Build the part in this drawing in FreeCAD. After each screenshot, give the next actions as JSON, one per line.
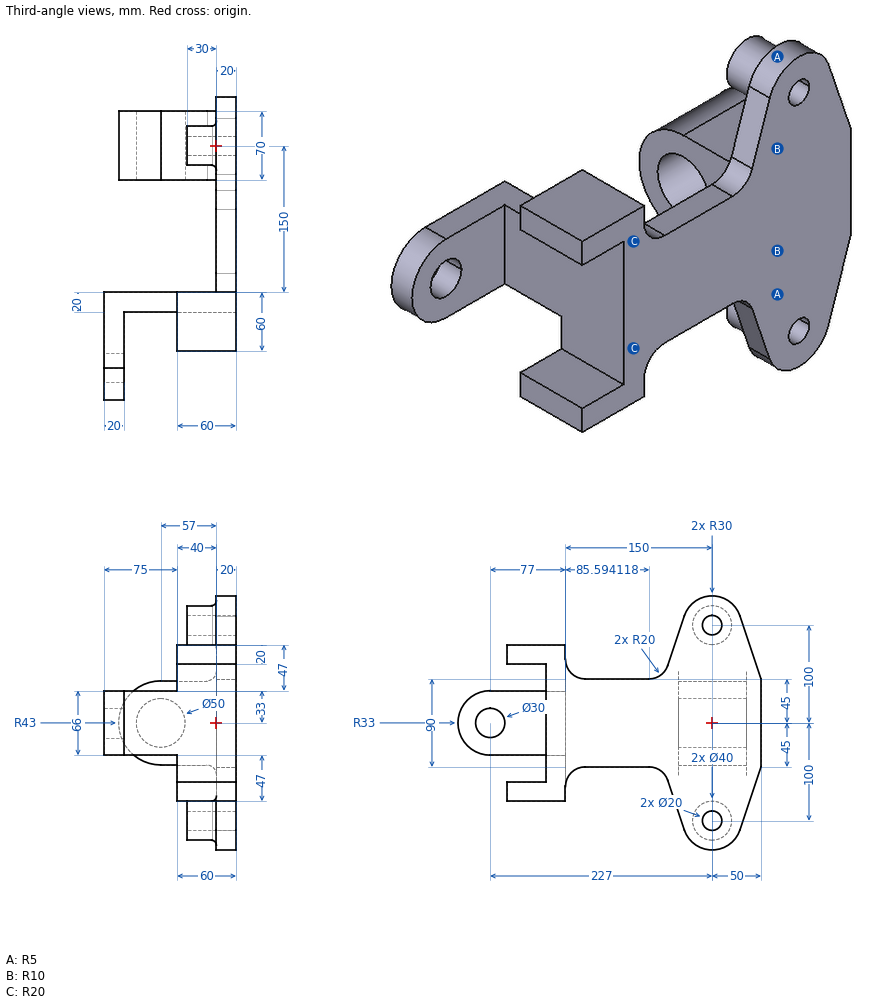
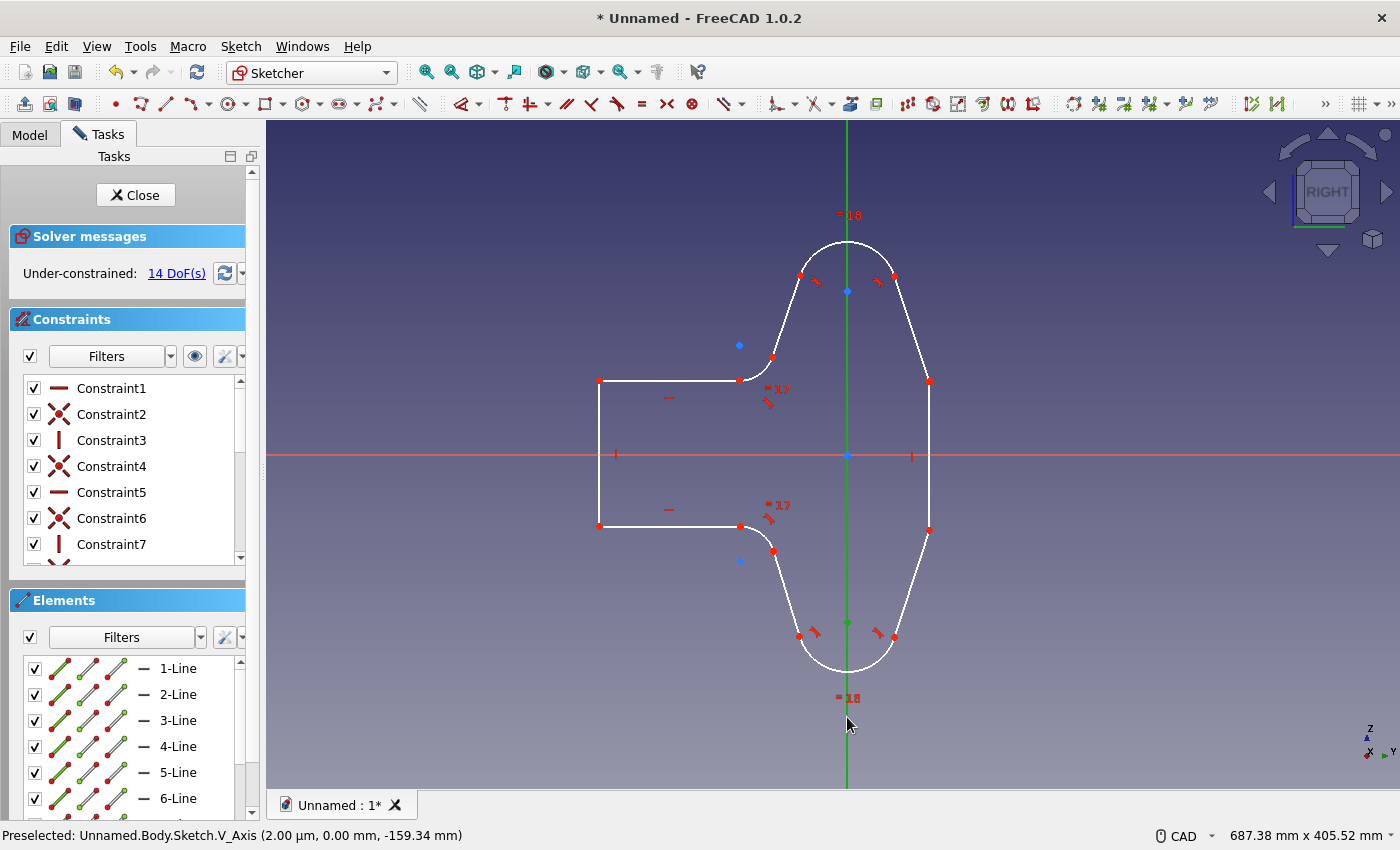
{"action": "left_click", "coordinate": [505, 104]}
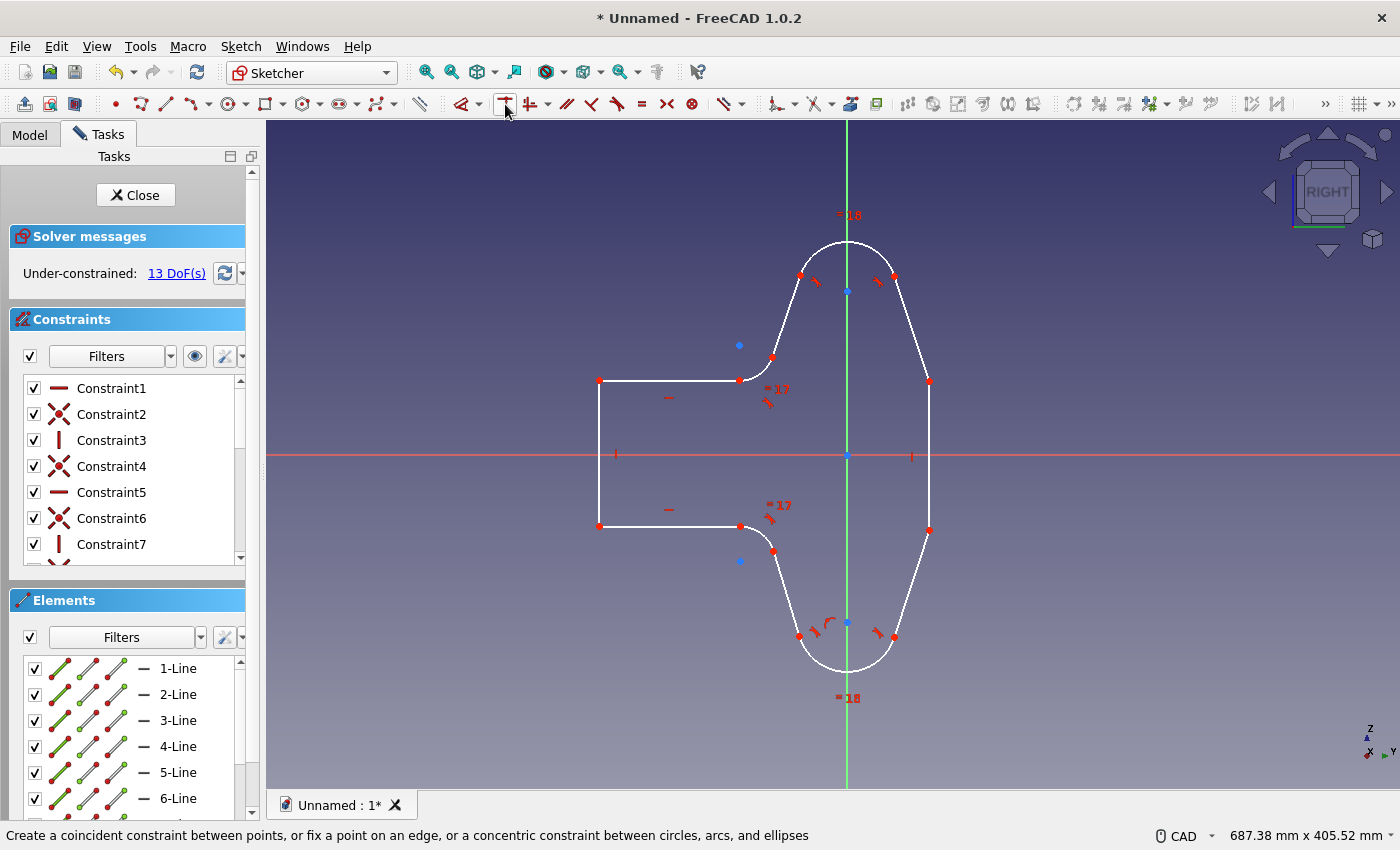
{"action": "left_click", "coordinate": [847, 292]}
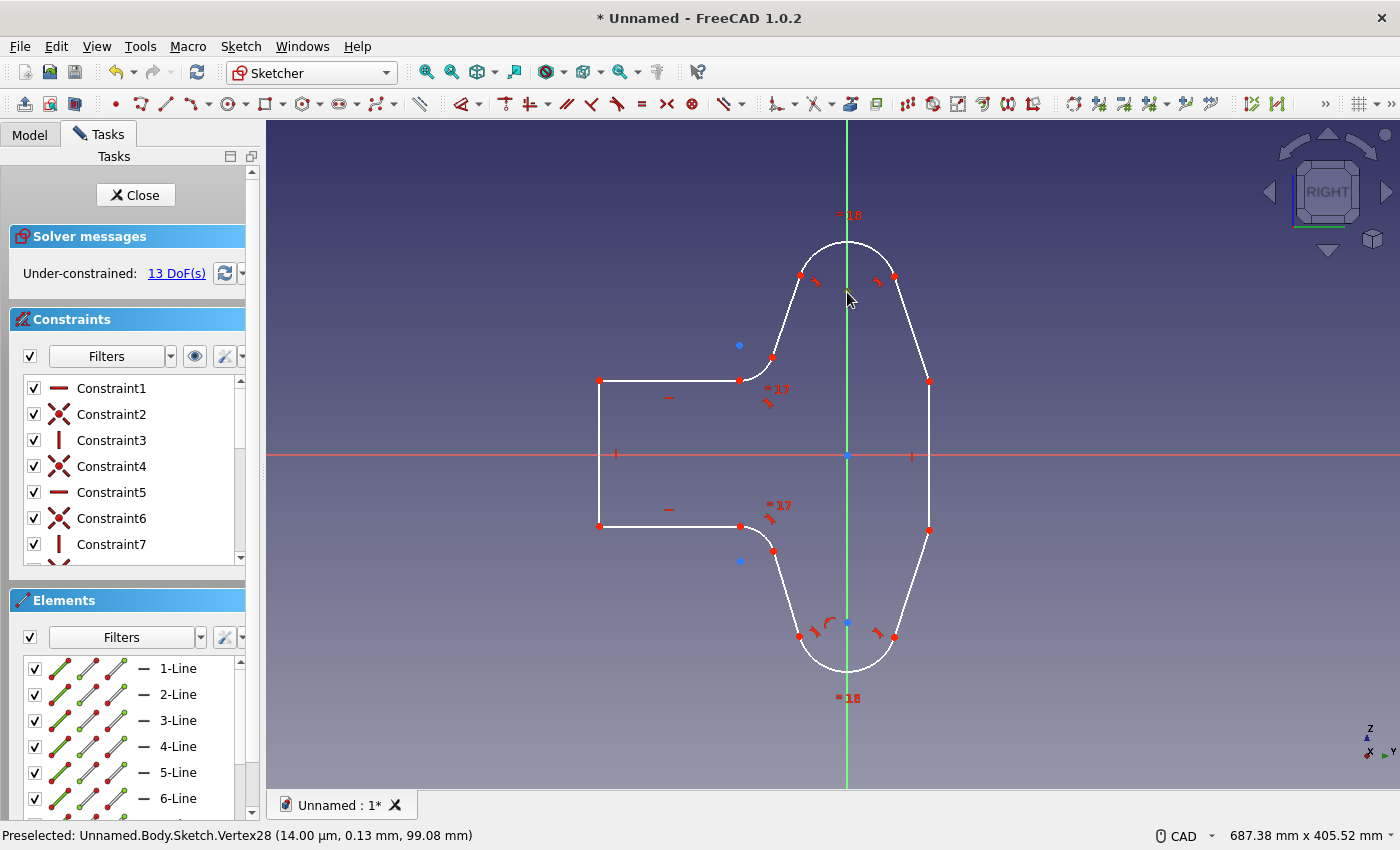
{"action": "left_click", "coordinate": [847, 717]}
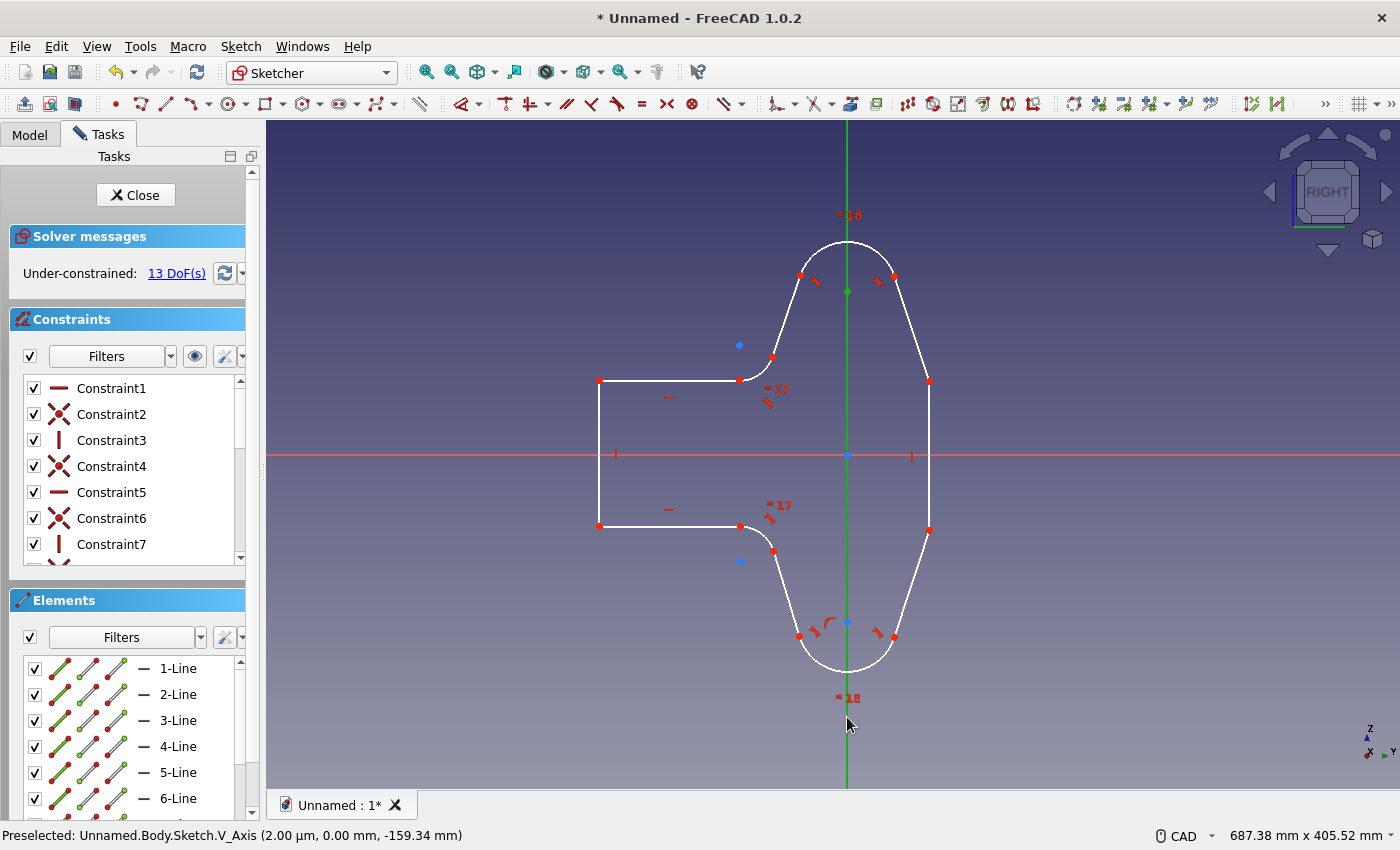
{"action": "left_click", "coordinate": [505, 104]}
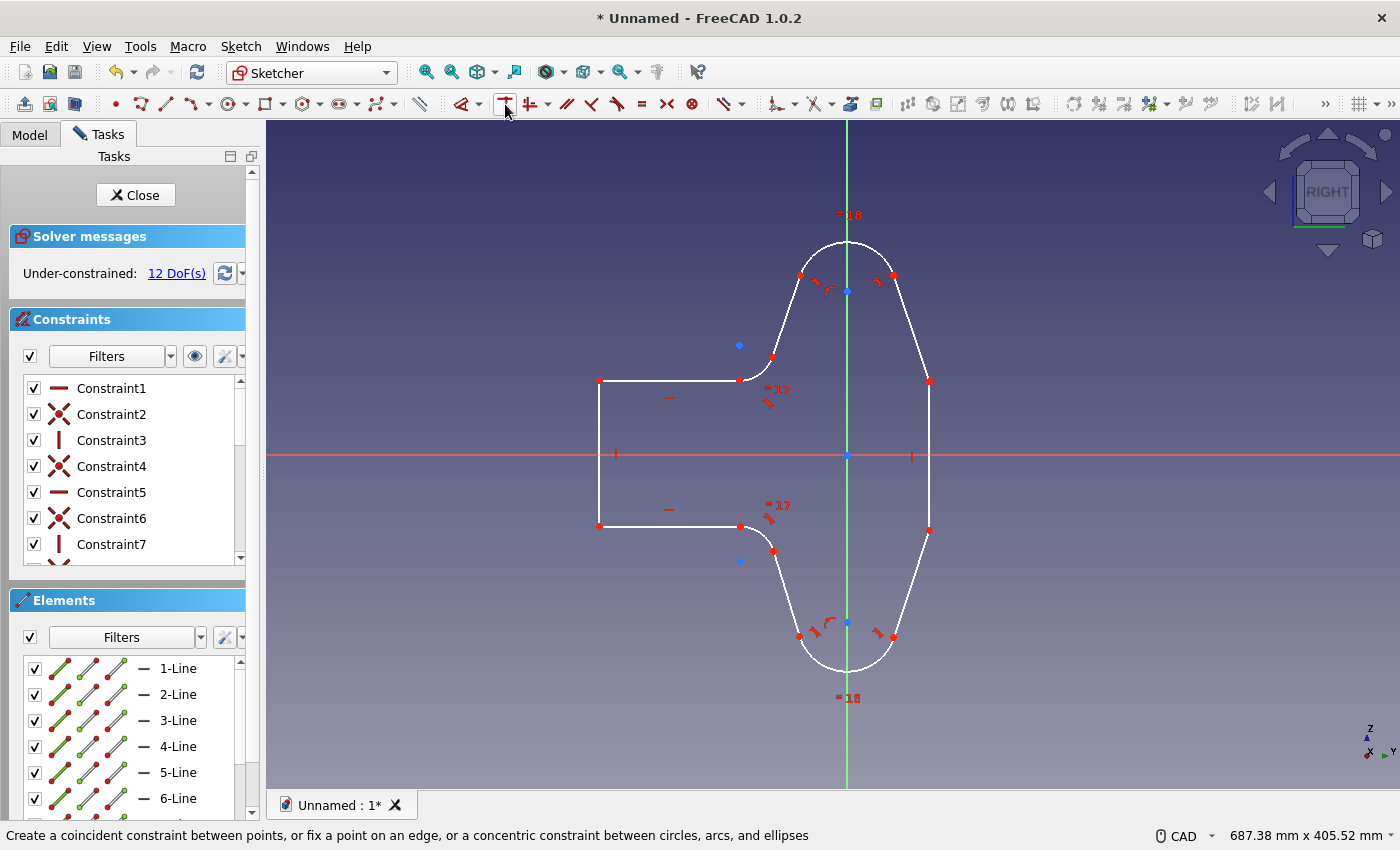
{"action": "left_click", "coordinate": [460, 104]}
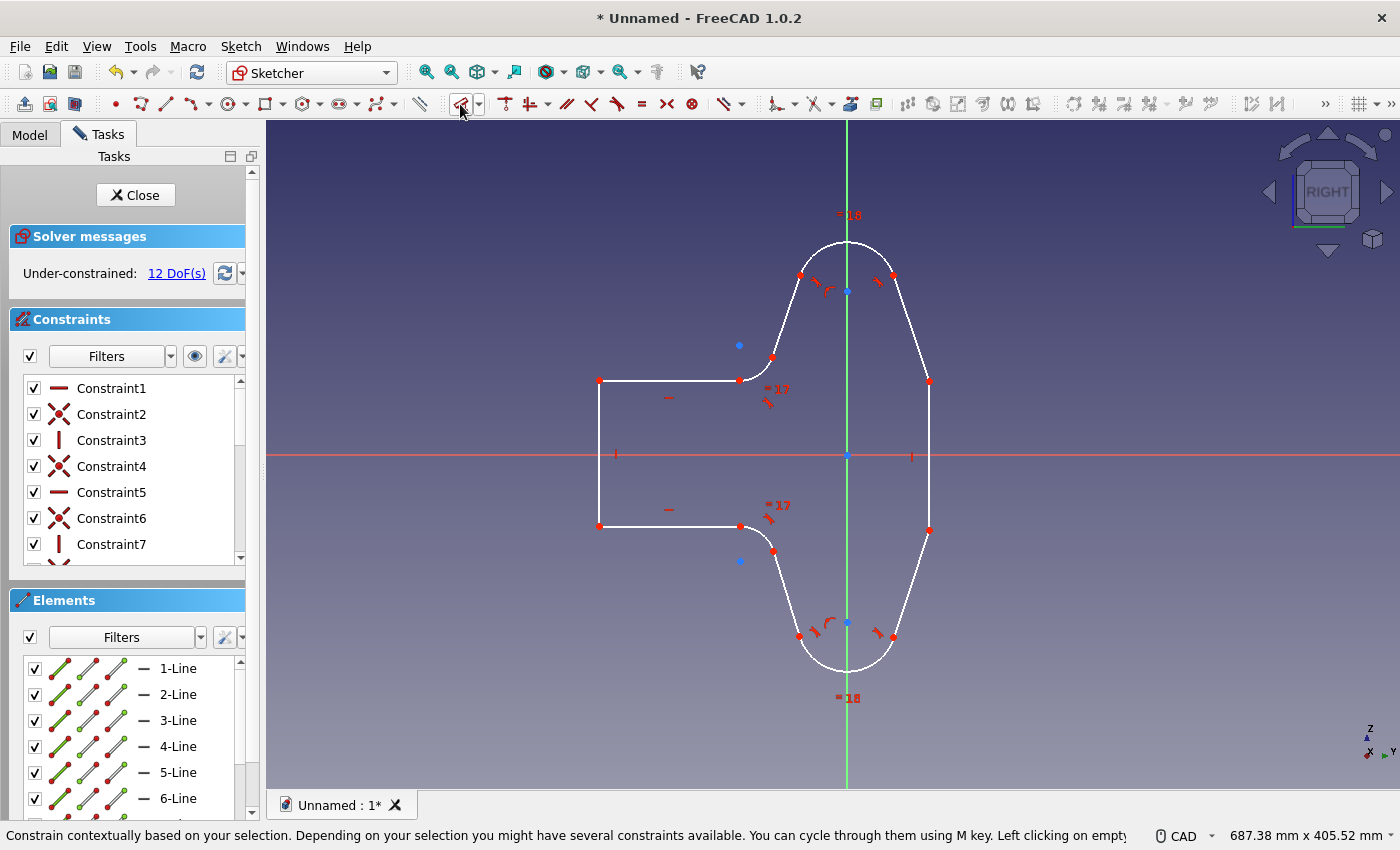
{"action": "left_click", "coordinate": [752, 378]}
{"action": "left_click", "coordinate": [764, 408]}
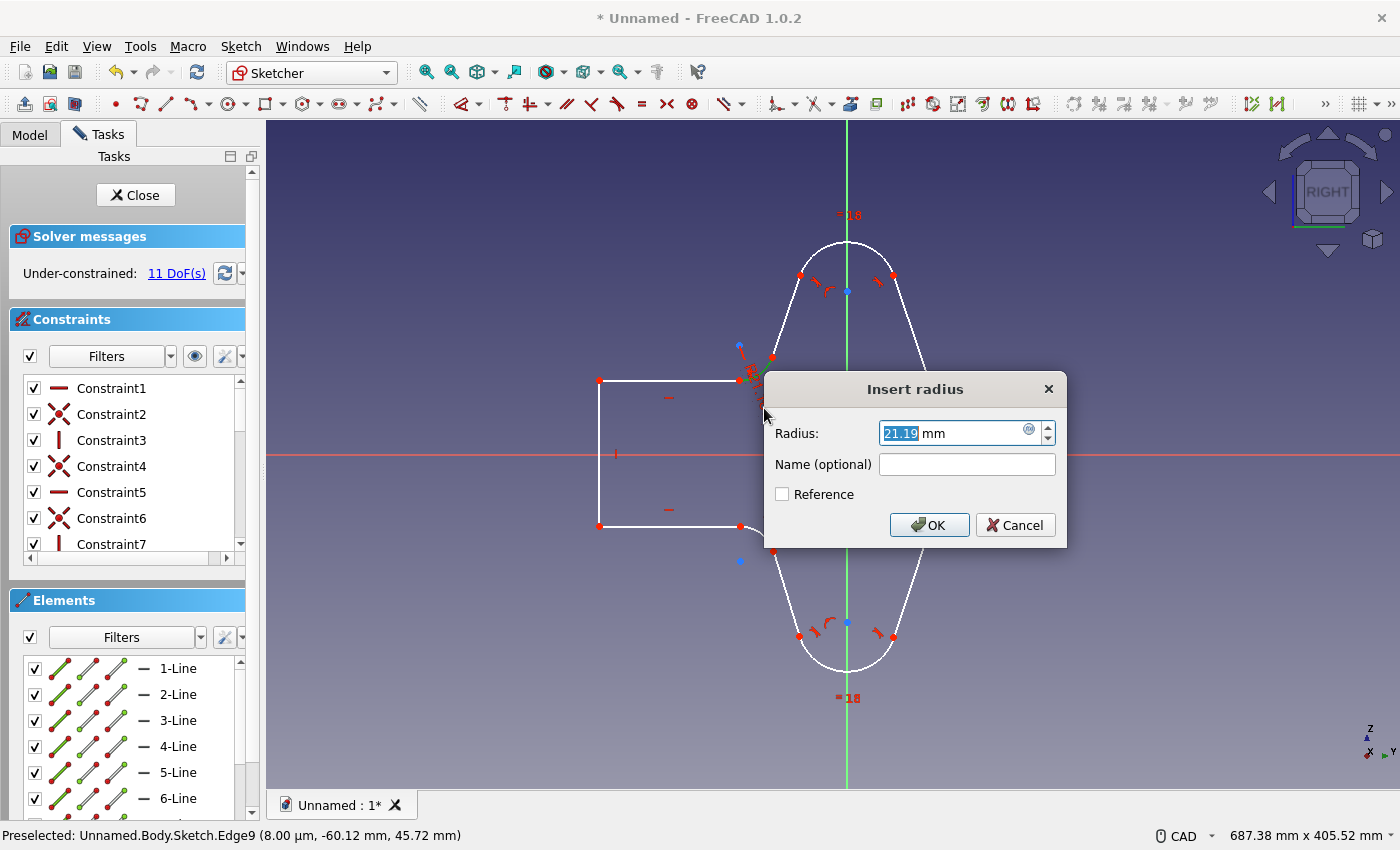
{"action": "type", "text": "20"}
{"action": "key", "text": "Return"}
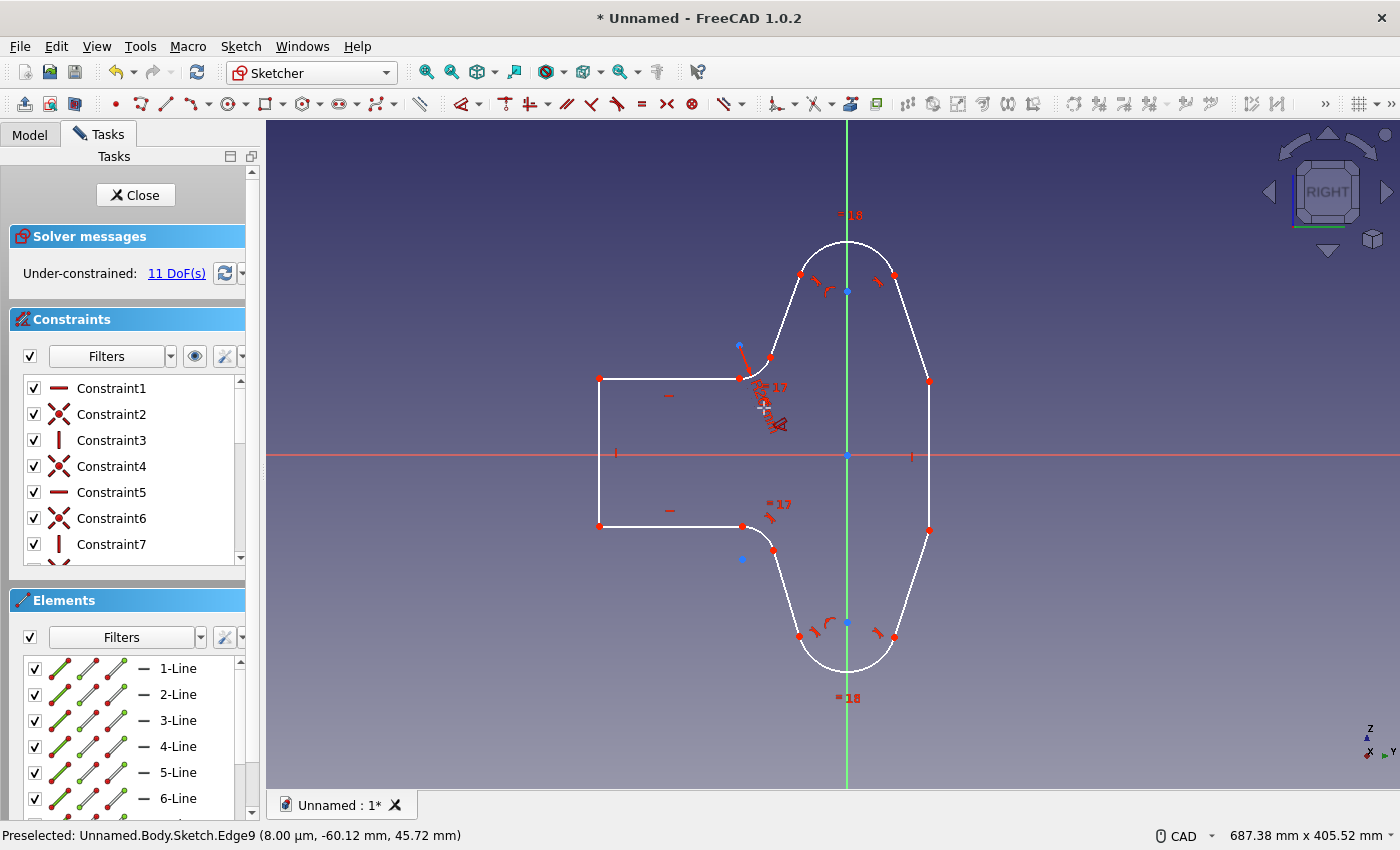
{"action": "left_click", "coordinate": [822, 665]}
{"action": "left_click", "coordinate": [806, 693]}